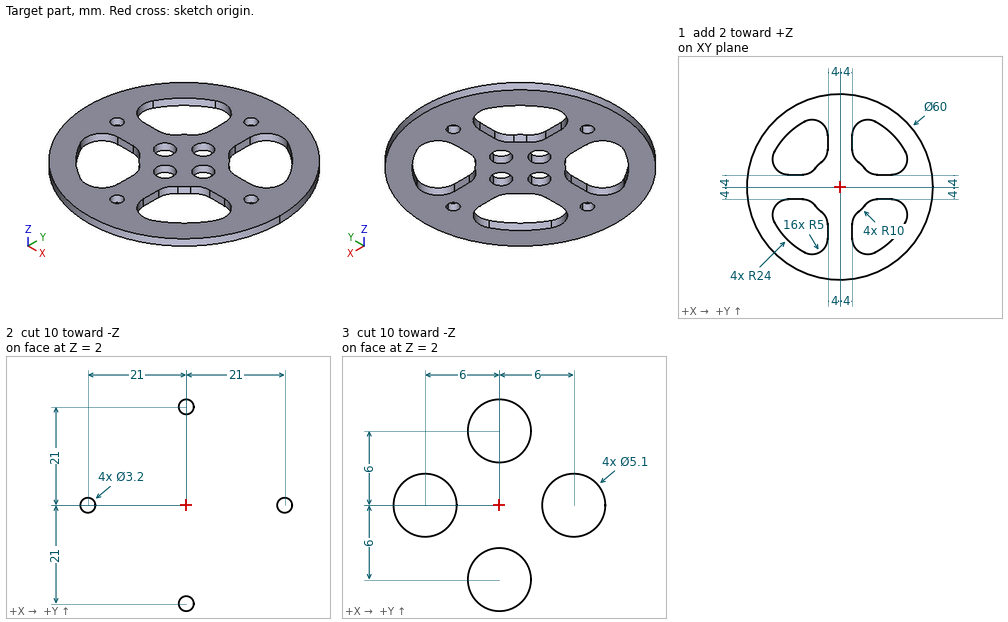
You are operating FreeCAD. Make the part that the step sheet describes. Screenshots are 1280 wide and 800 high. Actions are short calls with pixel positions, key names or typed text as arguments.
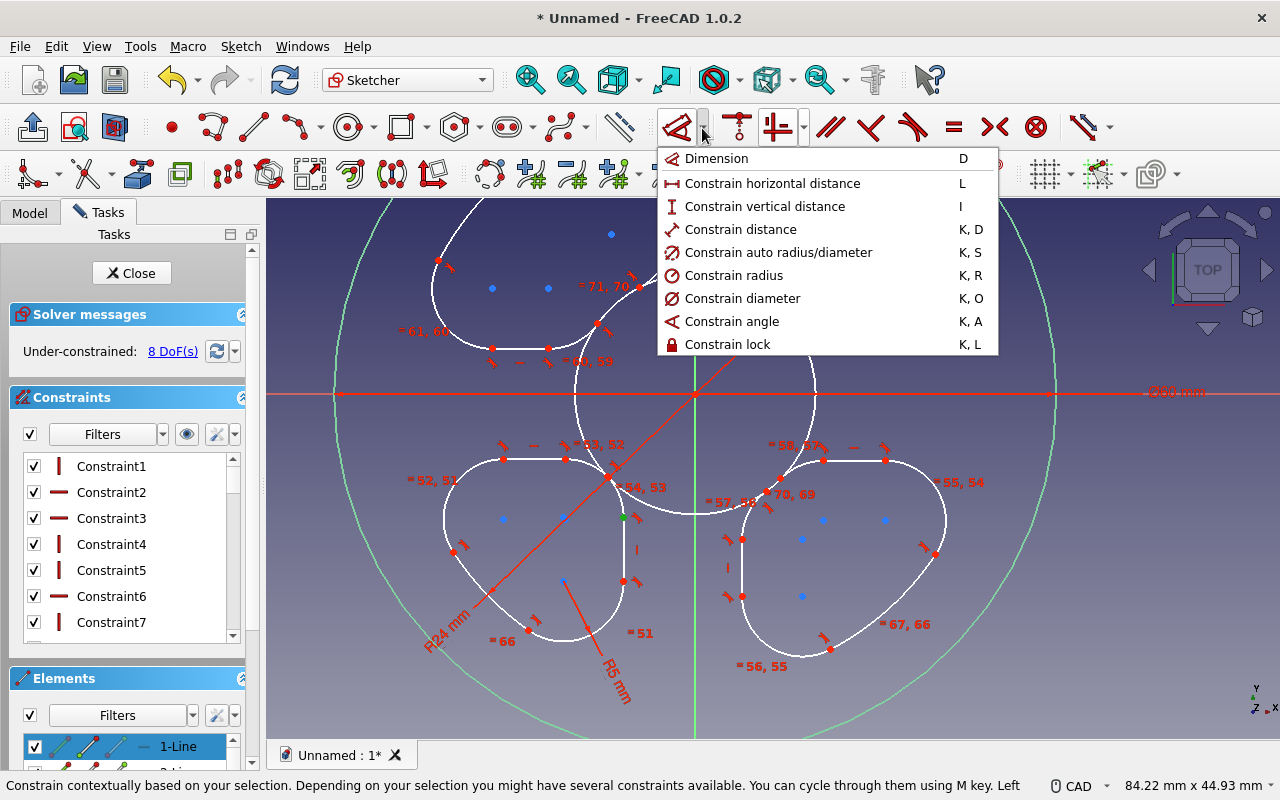
click(828, 184)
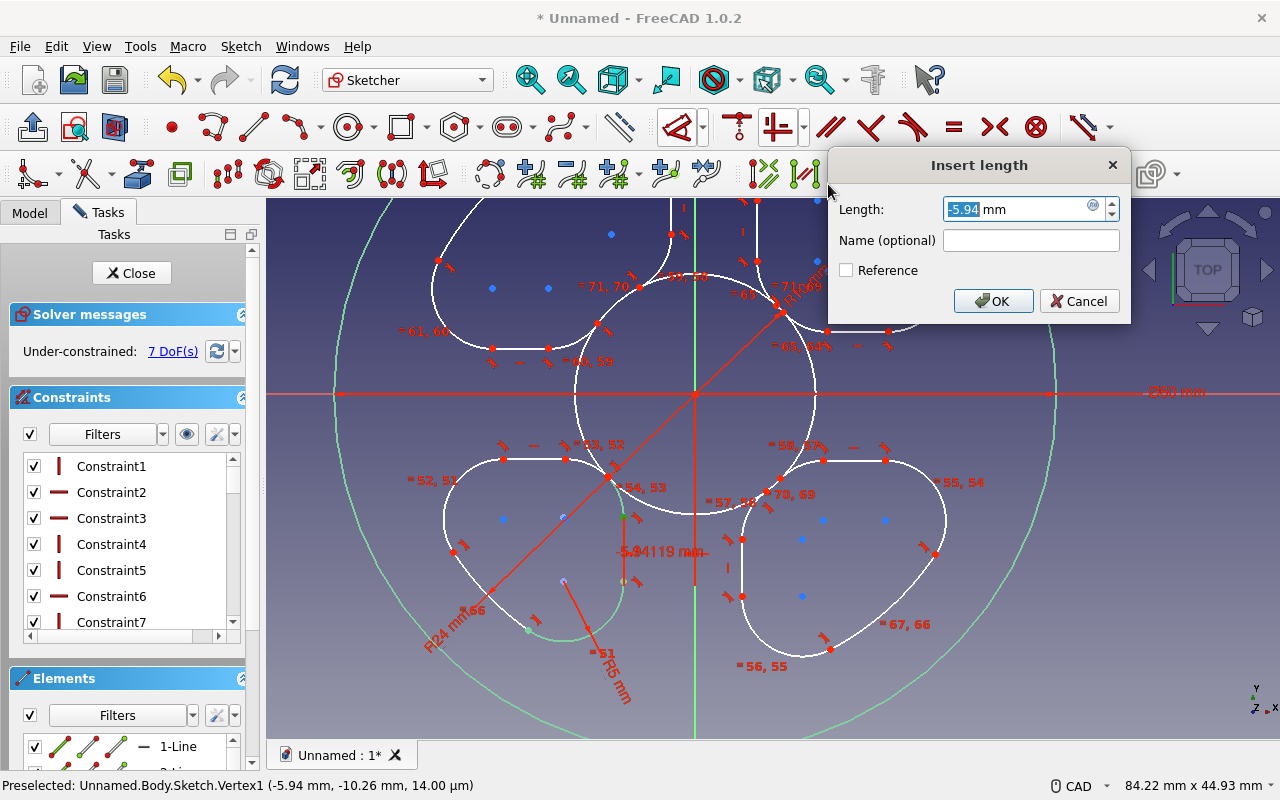
text(-4)
key(Return)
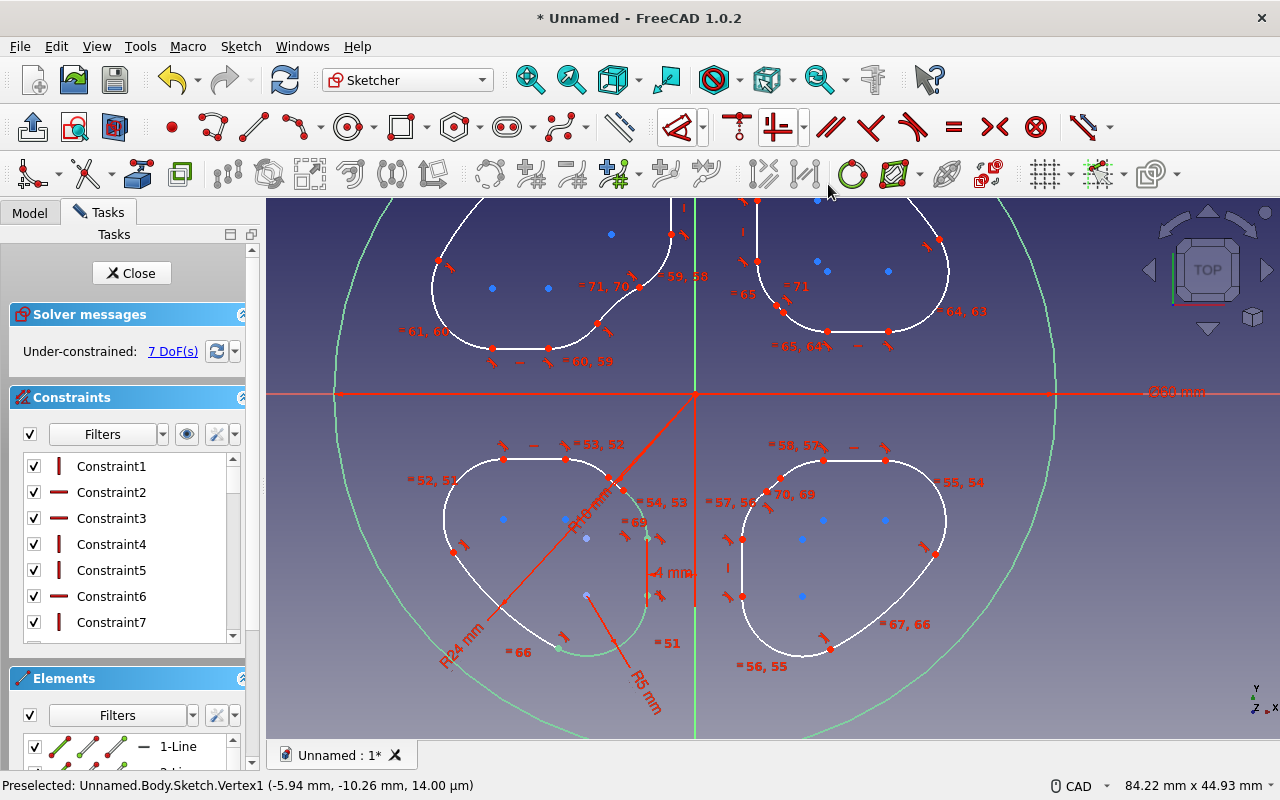
click(504, 459)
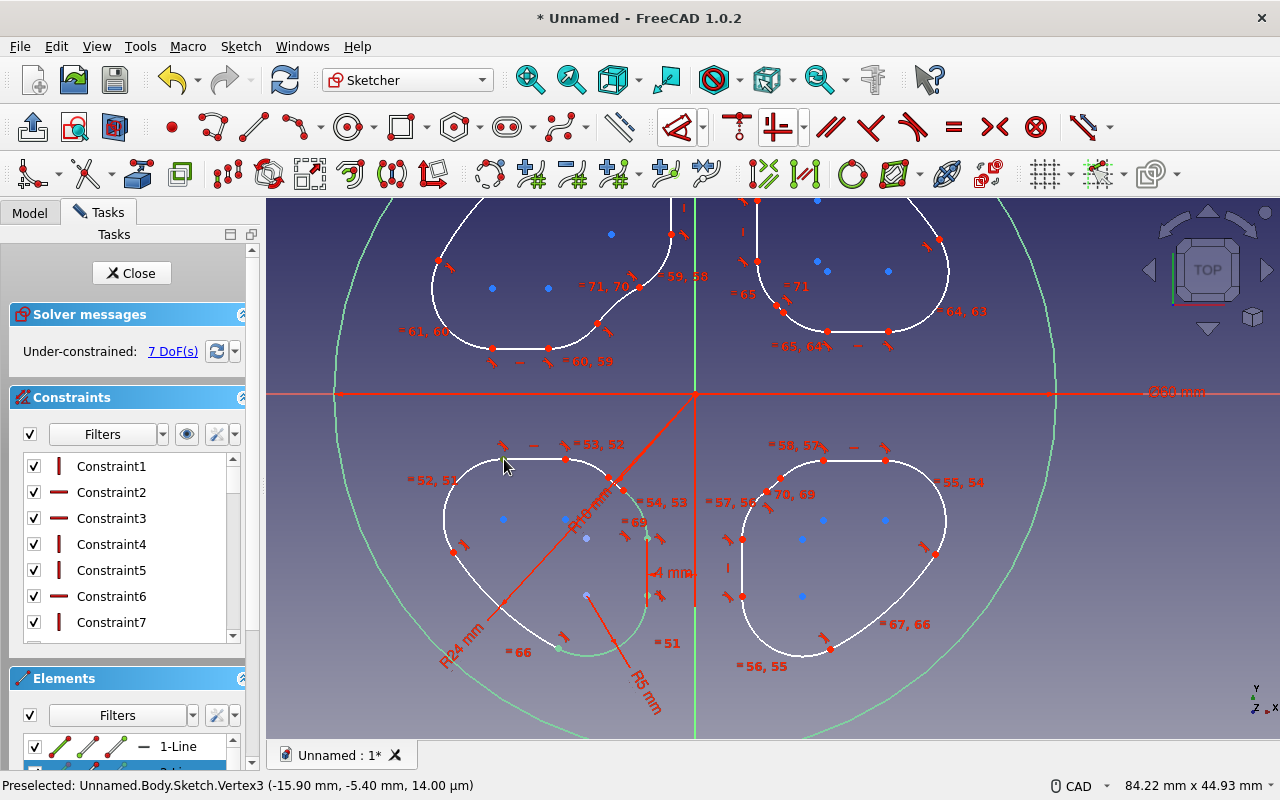
key(i)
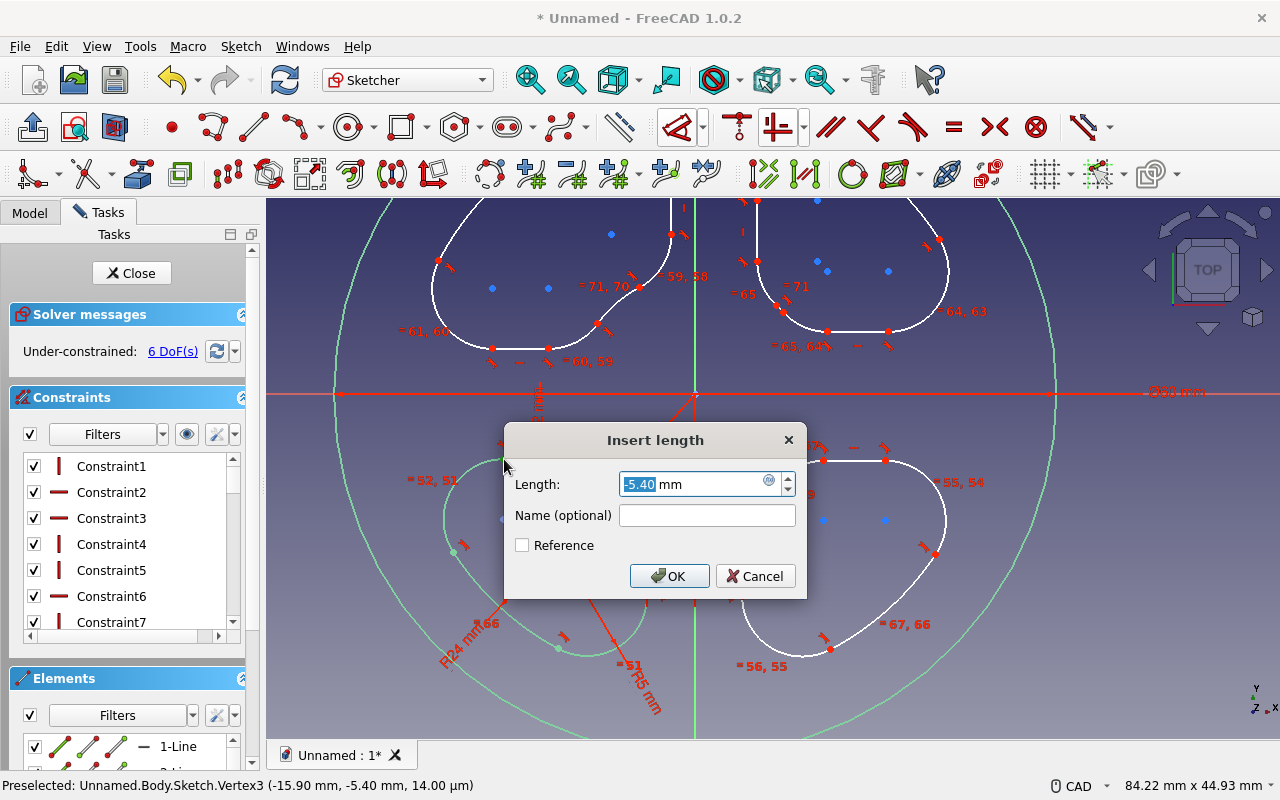
text(-4)
key(Return)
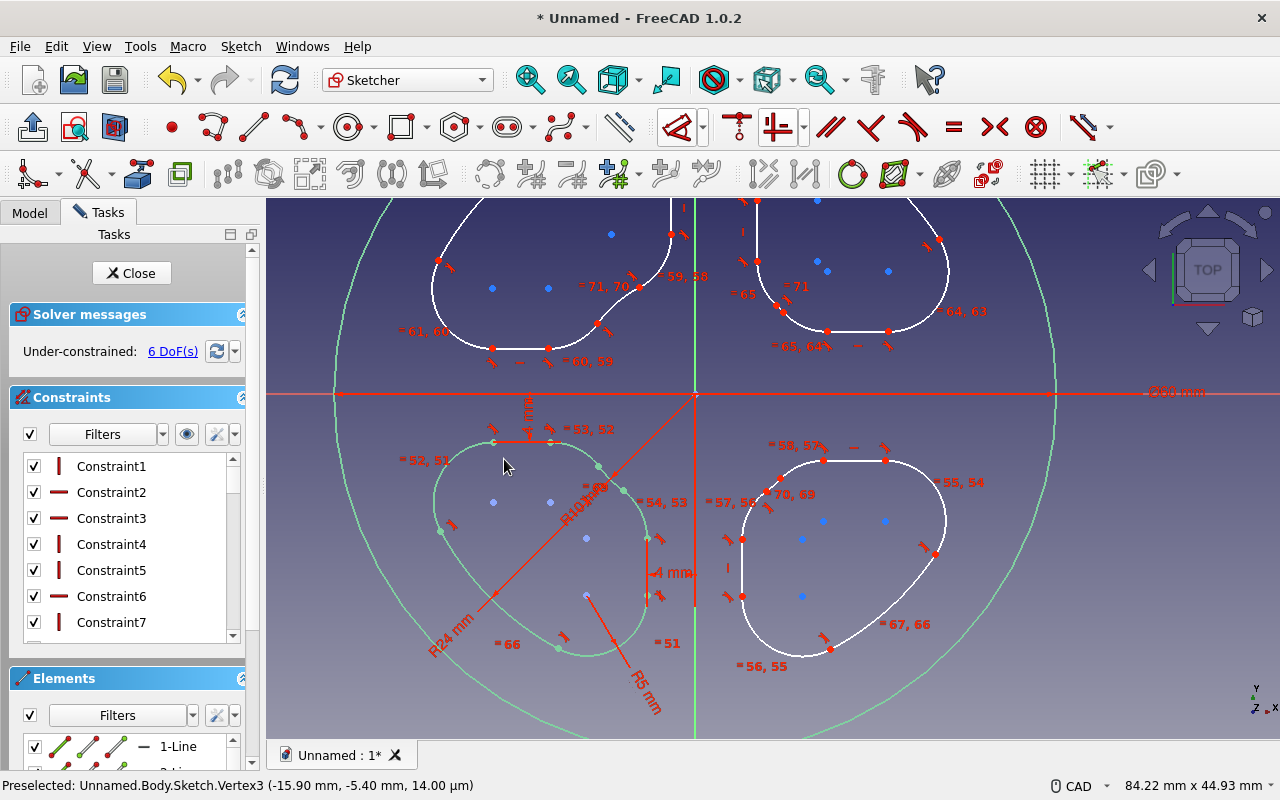
click(824, 461)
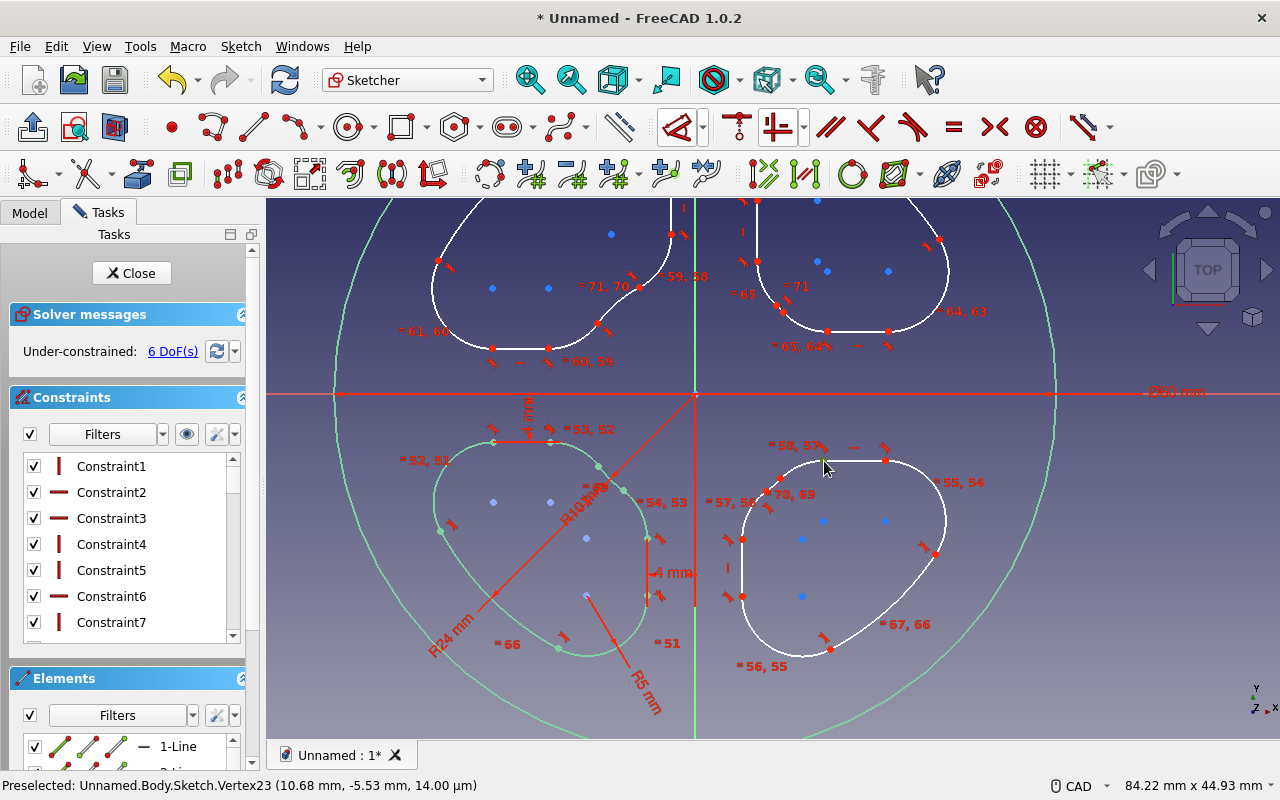
key(i)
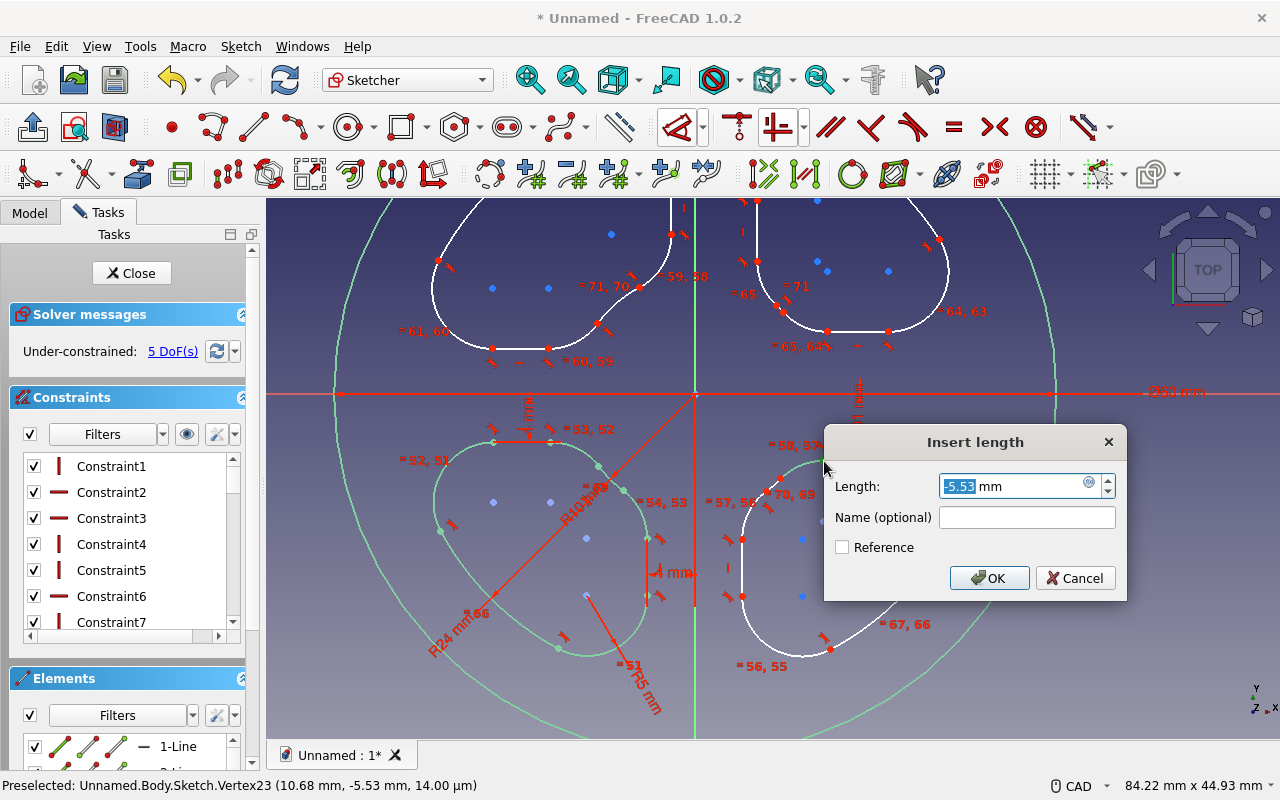
text(-4)
key(Return)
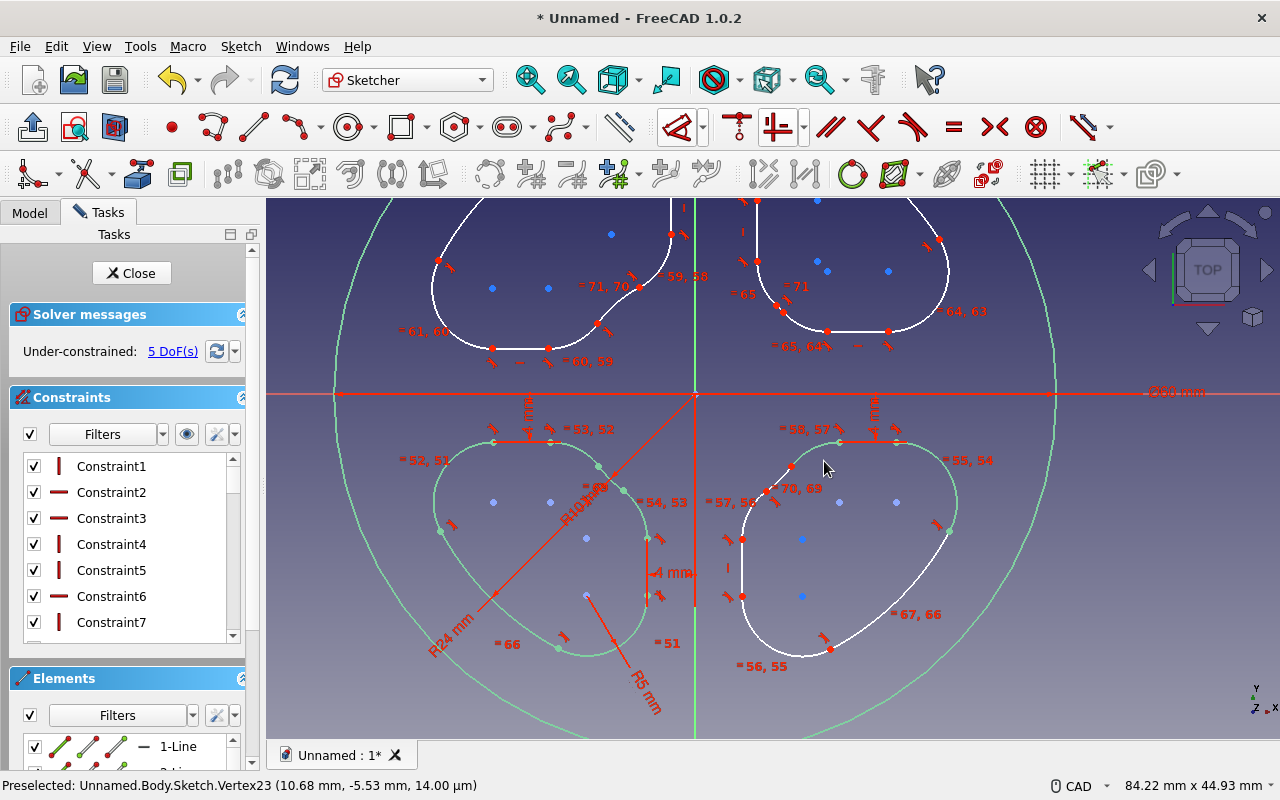
click(742, 596)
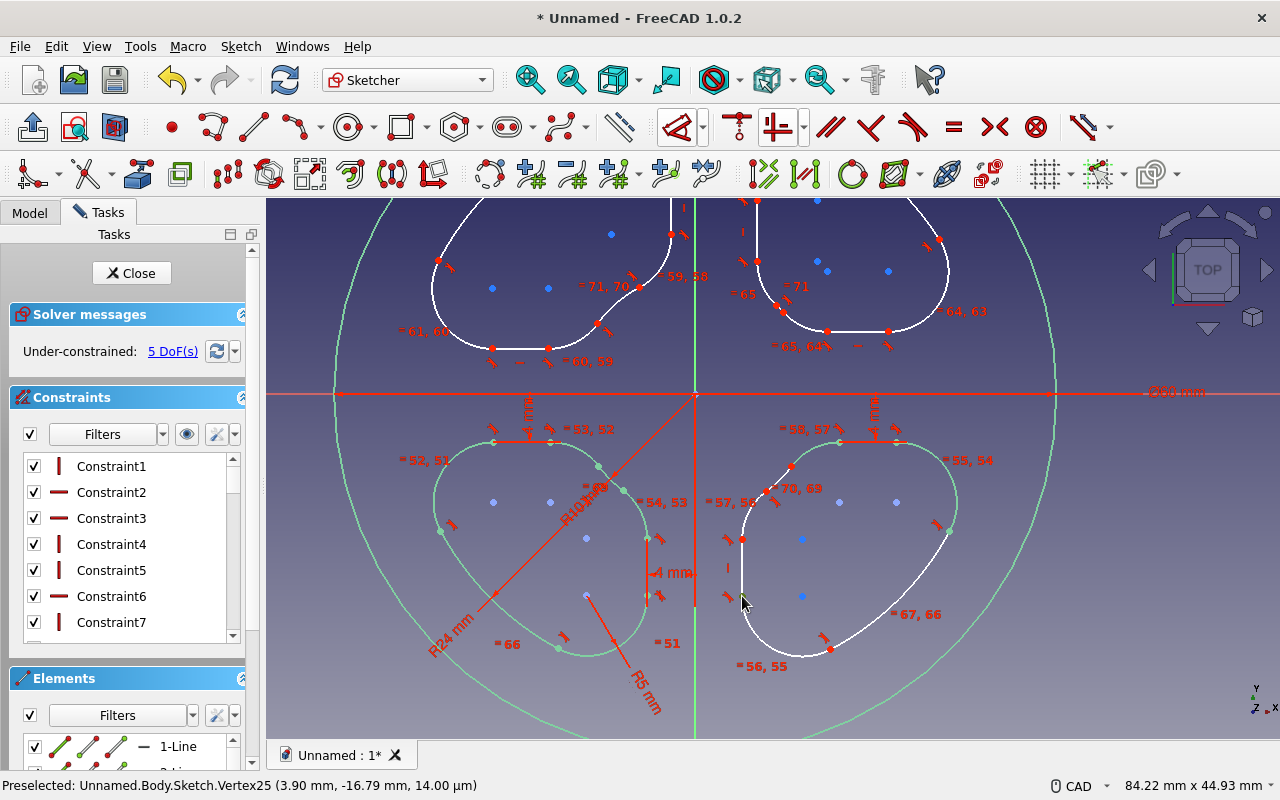
click(702, 128)